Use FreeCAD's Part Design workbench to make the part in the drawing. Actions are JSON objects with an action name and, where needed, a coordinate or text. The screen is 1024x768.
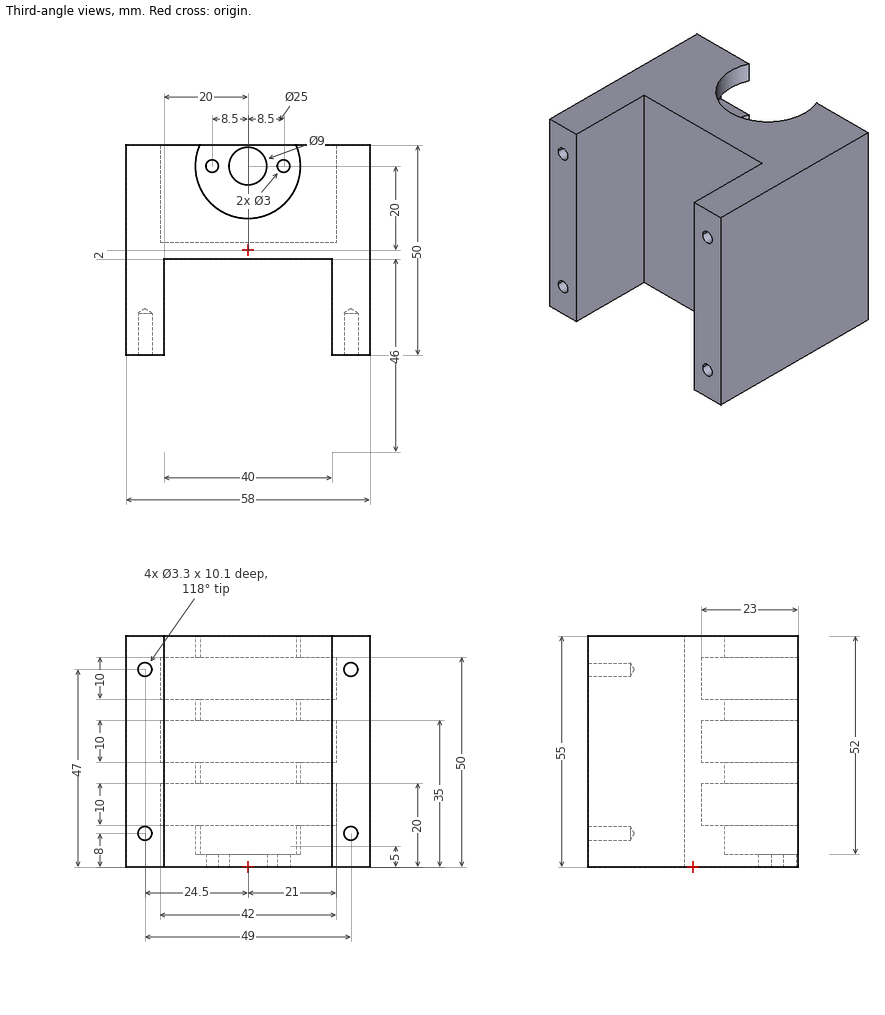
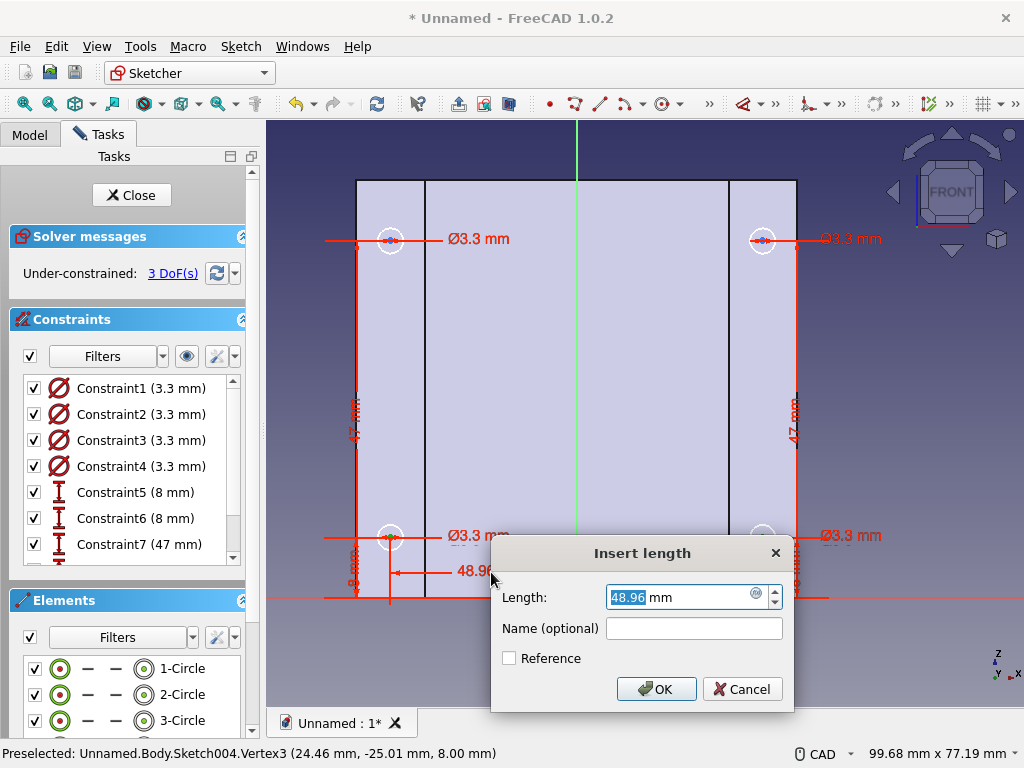
{"action": "type", "text": "49"}
{"action": "key", "text": "Return"}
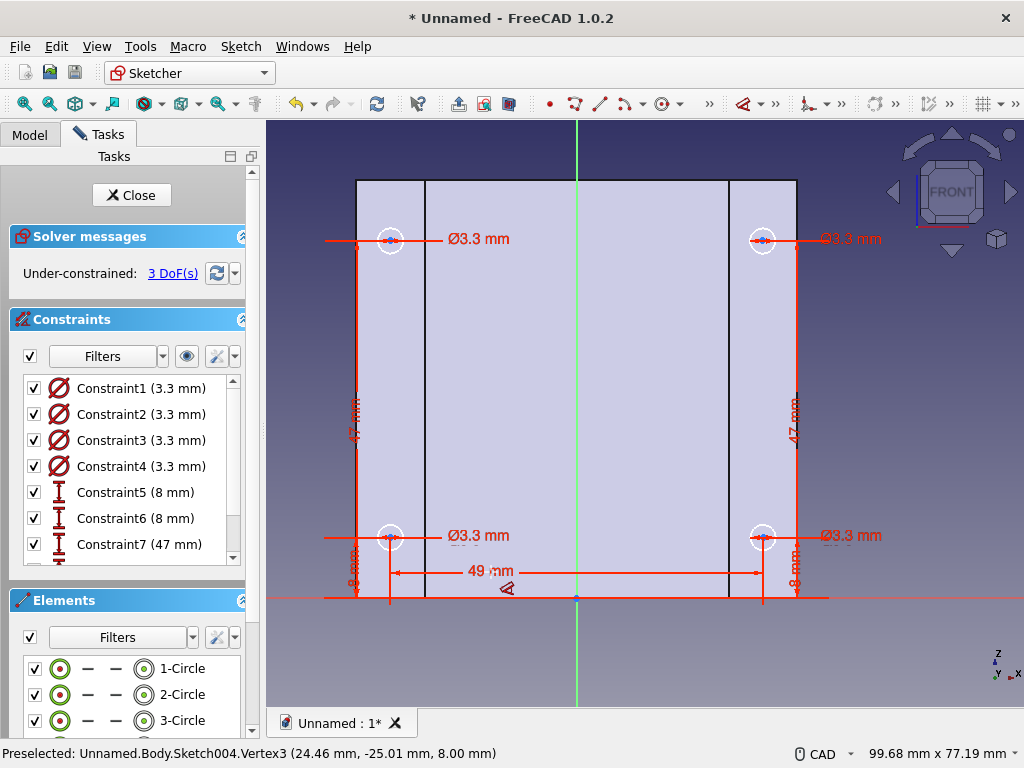
{"action": "left_click", "coordinate": [391, 241]}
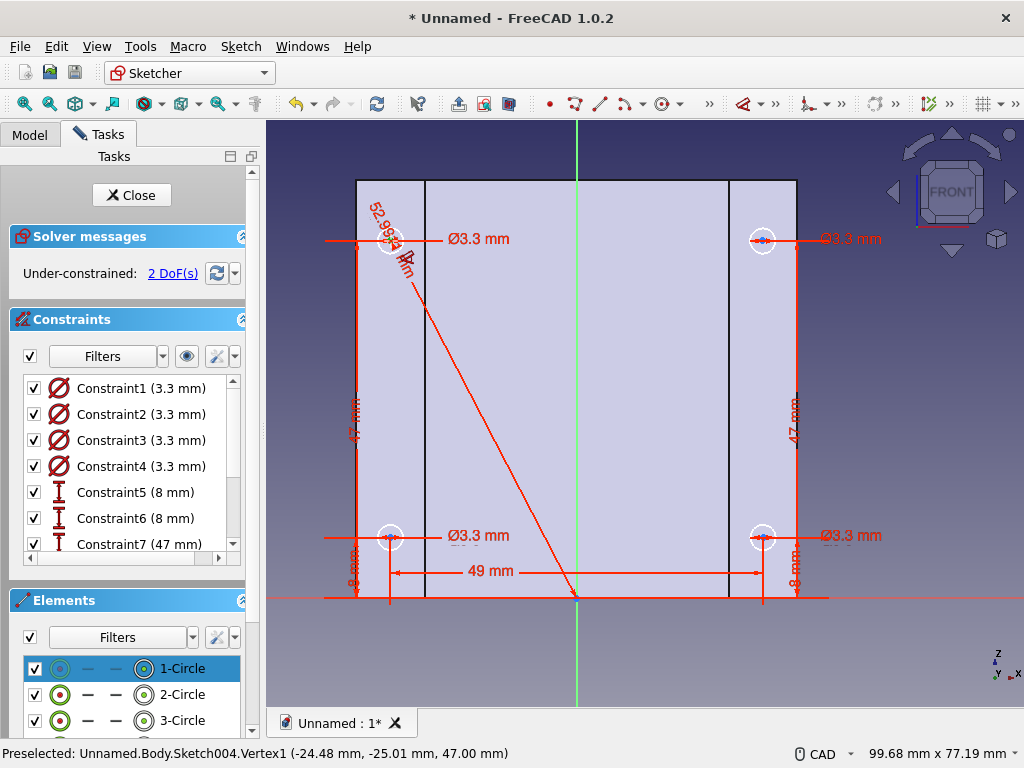
{"action": "left_click", "coordinate": [763, 538]}
{"action": "left_click", "coordinate": [491, 207]}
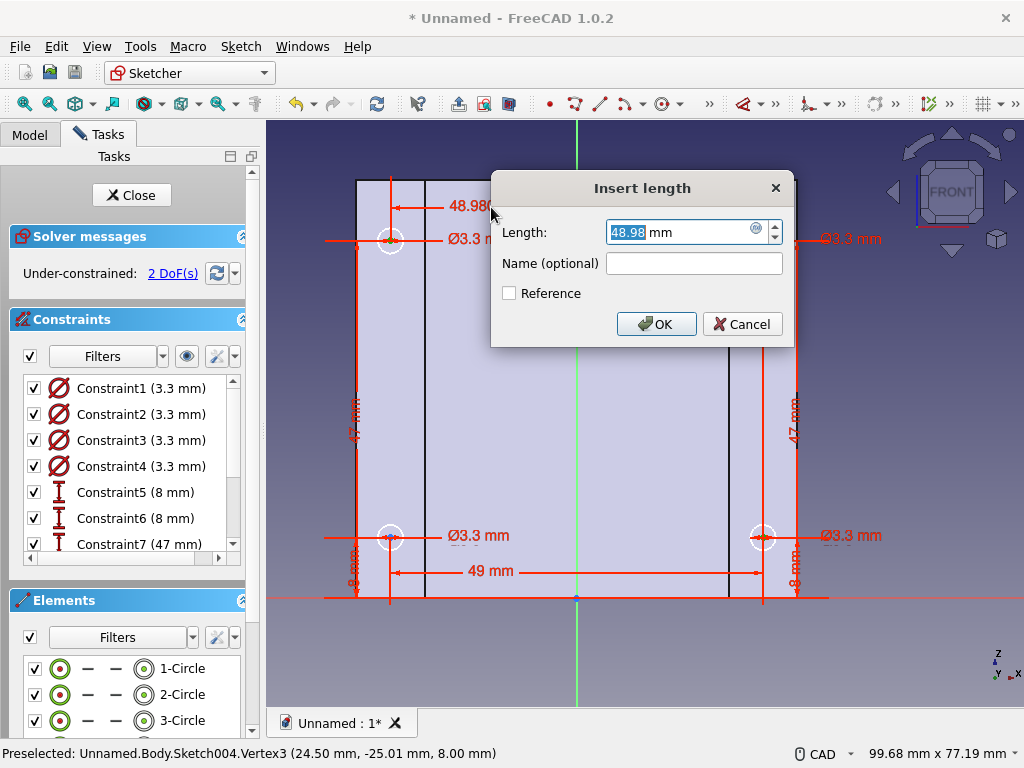
{"action": "type", "text": "49"}
{"action": "key", "text": "Return"}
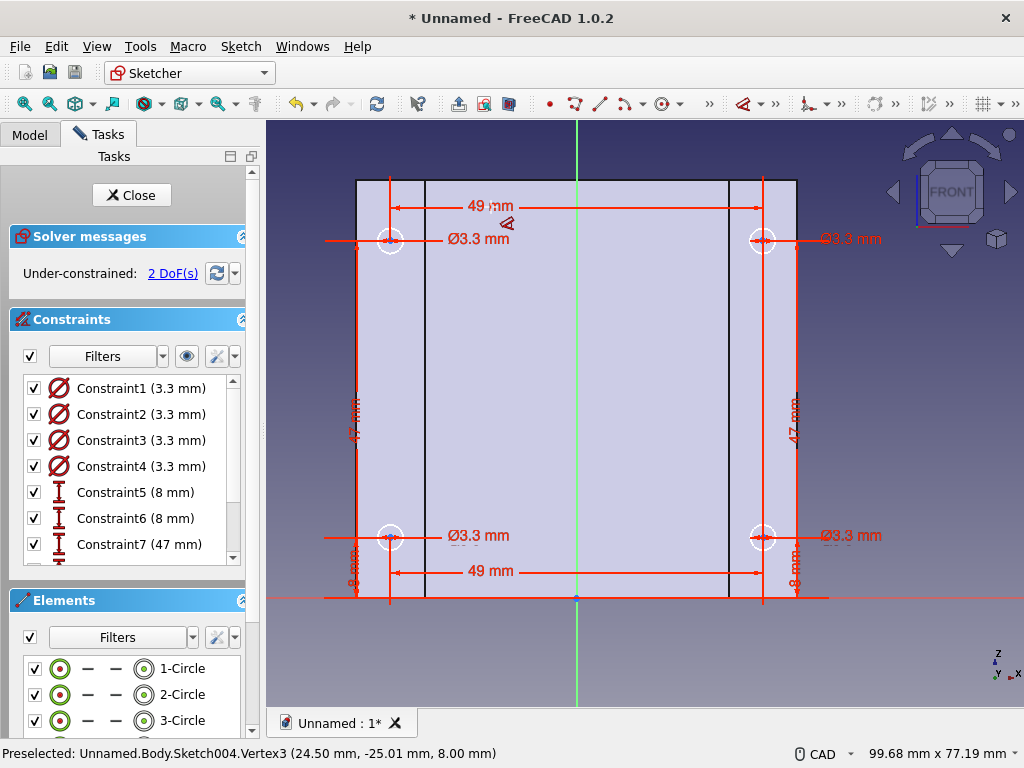
{"action": "left_click", "coordinate": [390, 241]}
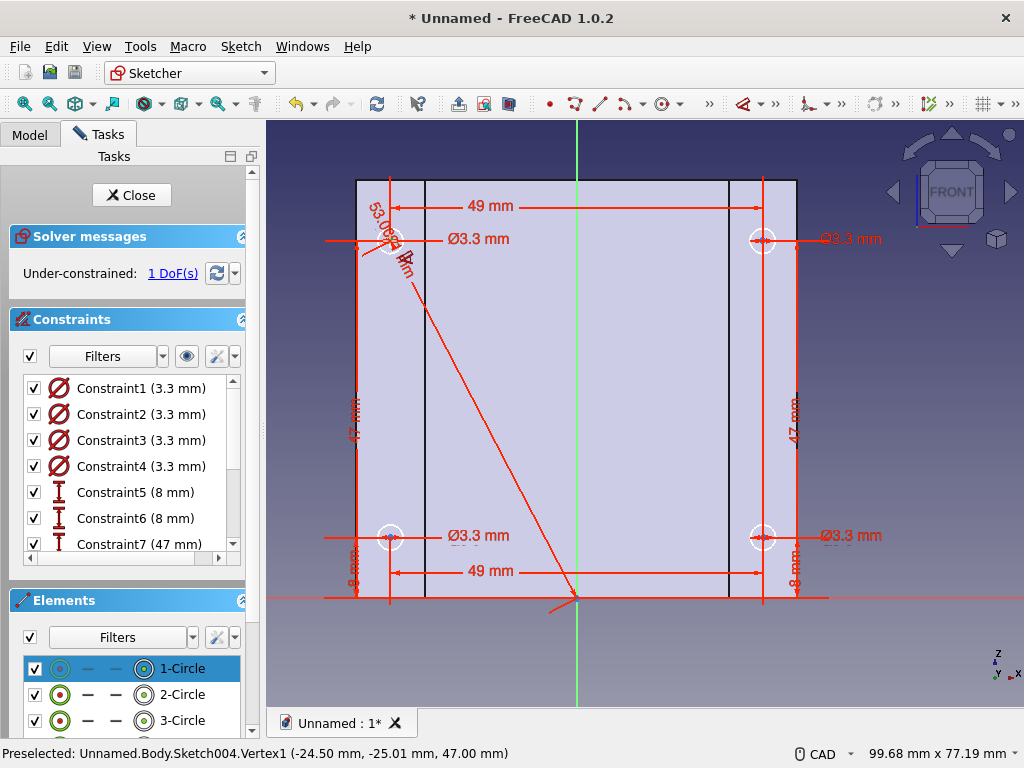
{"action": "left_click", "coordinate": [763, 241]}
{"action": "left_click", "coordinate": [662, 207]}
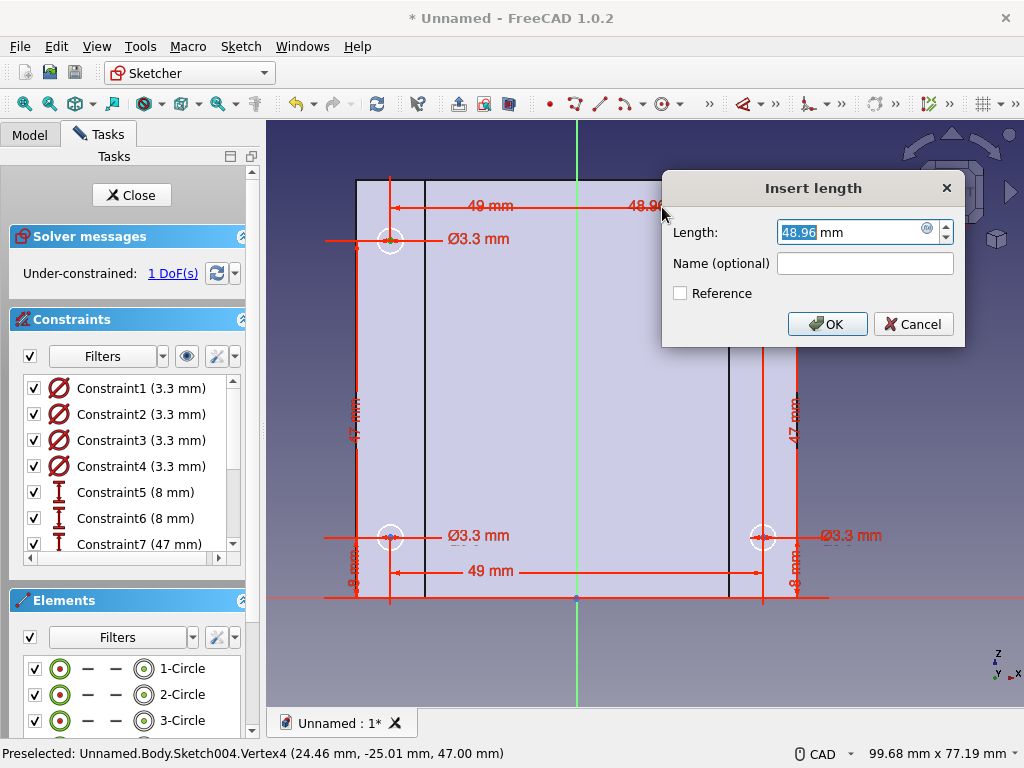
{"action": "type", "text": "49"}
{"action": "key", "text": "Return"}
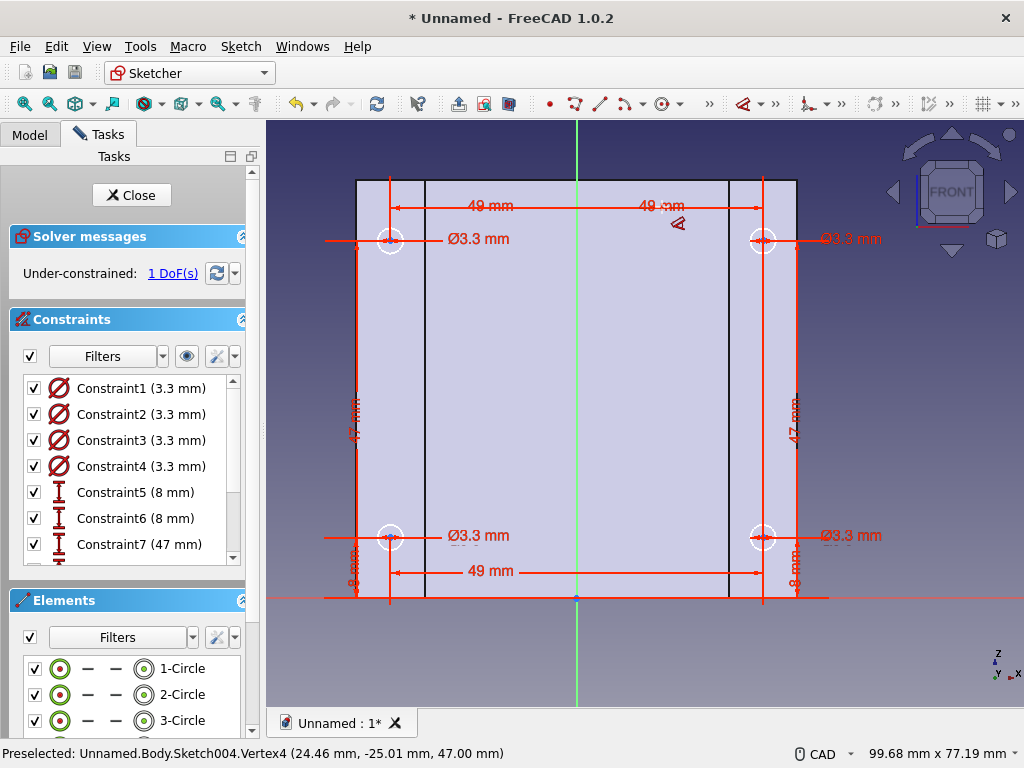
{"action": "left_click", "coordinate": [390, 241]}
{"action": "left_click", "coordinate": [484, 632]}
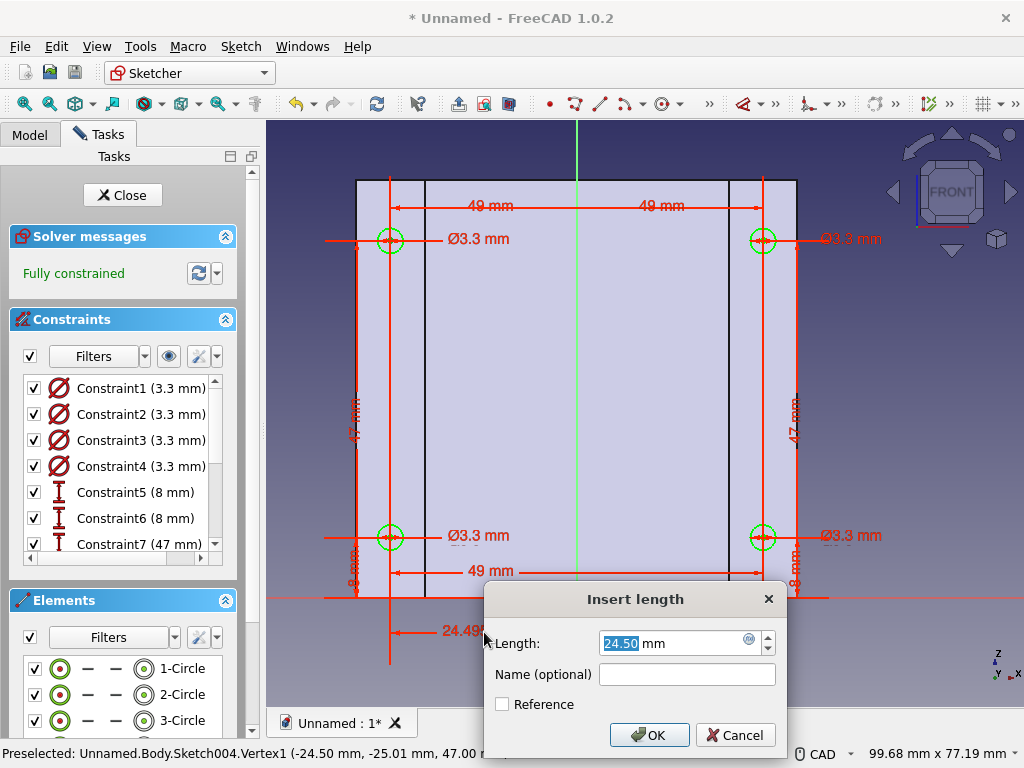
{"action": "type", "text": "24.5"}
{"action": "key", "text": "Return"}
{"action": "key", "text": "Escape"}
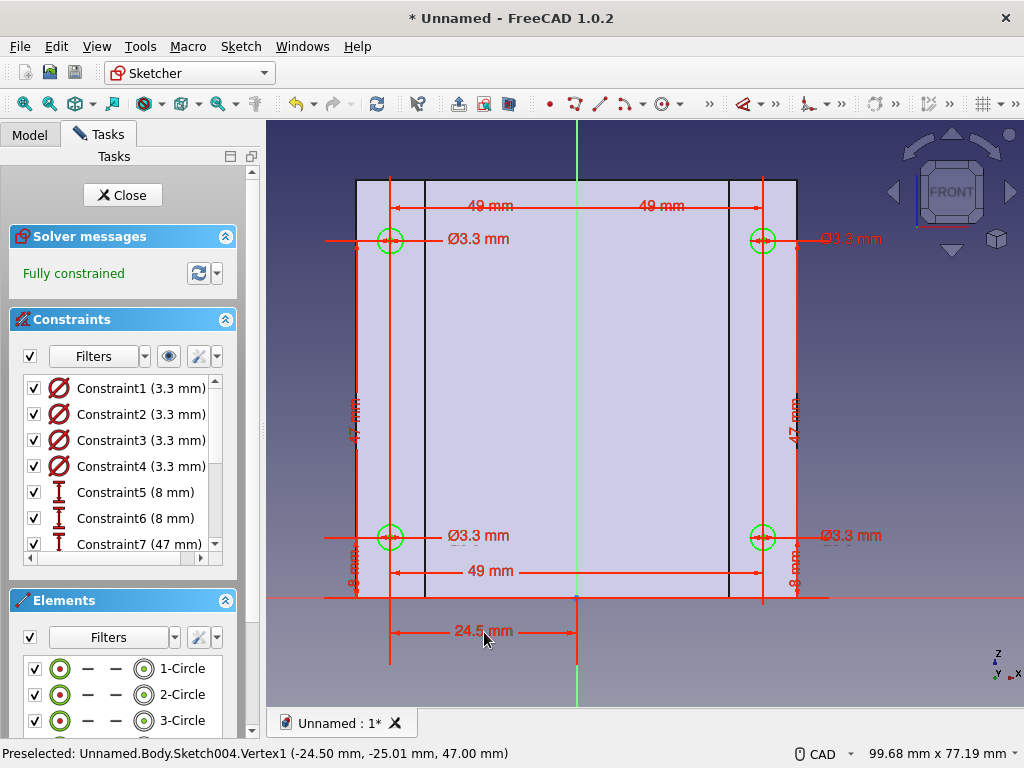
{"action": "left_click", "coordinate": [123, 195]}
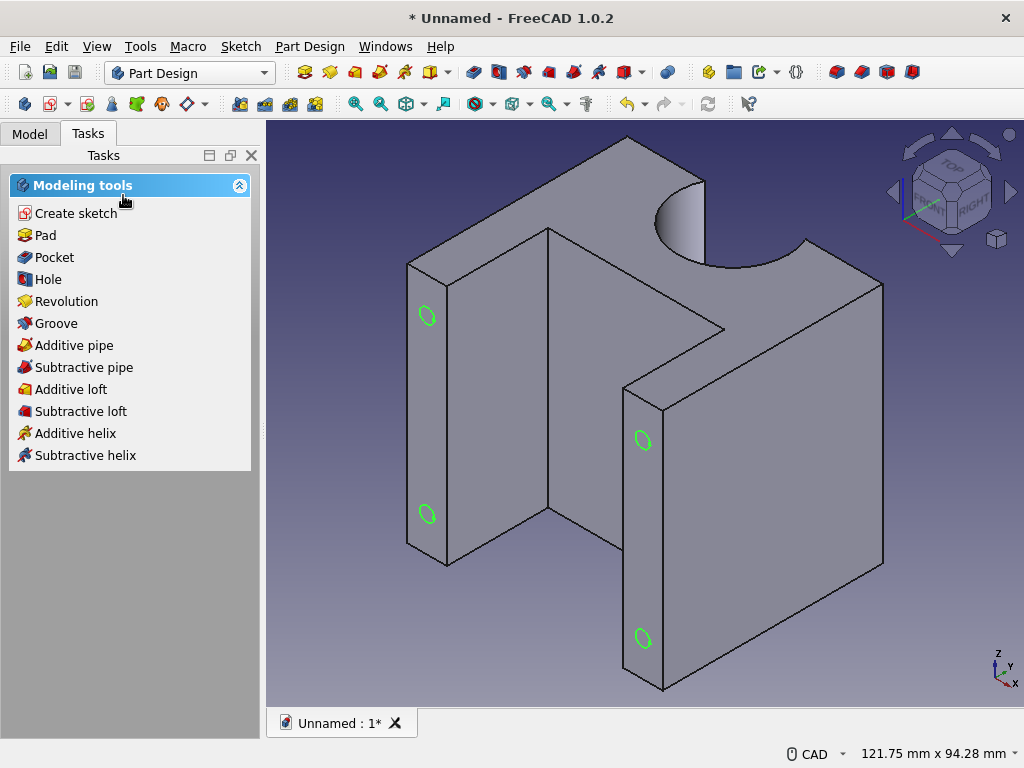
{"action": "left_click", "coordinate": [499, 72]}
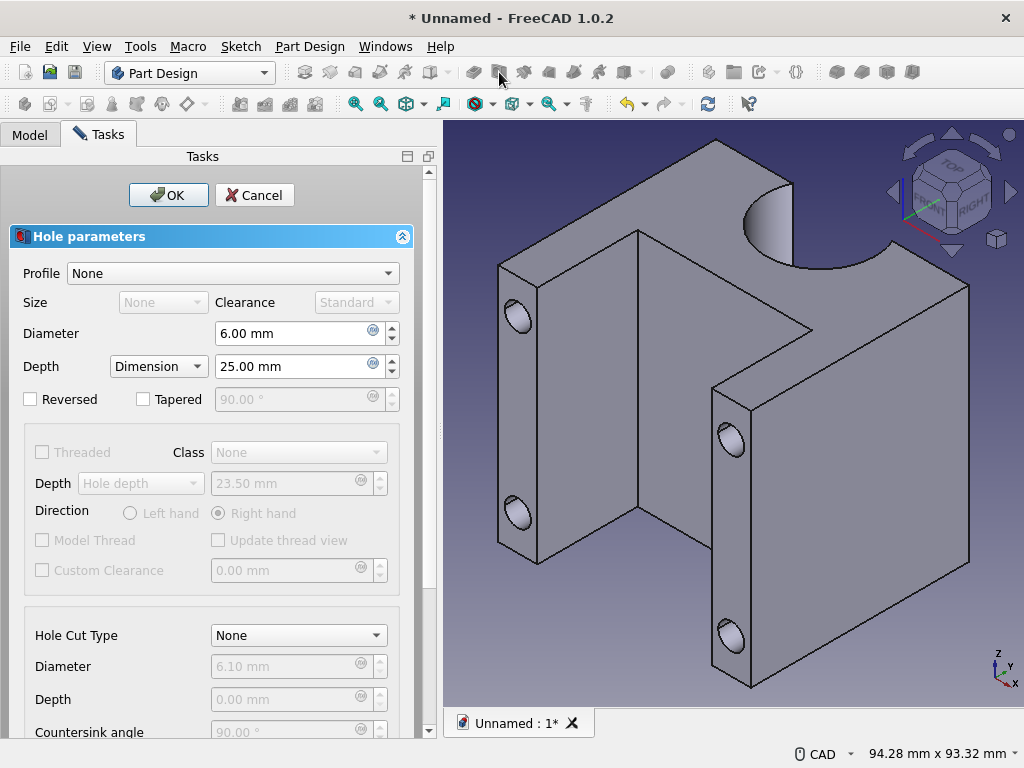
{"action": "triple_click", "coordinate": [300, 334]}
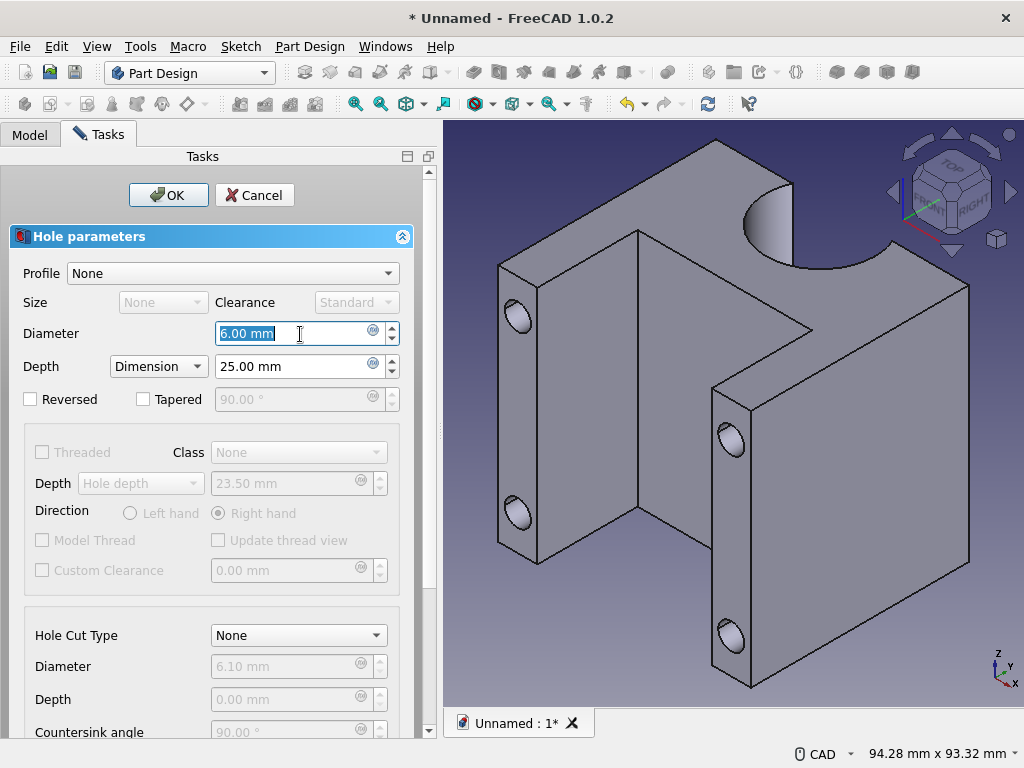
{"action": "type", "text": "3.3"}
{"action": "key", "text": "Tab"}